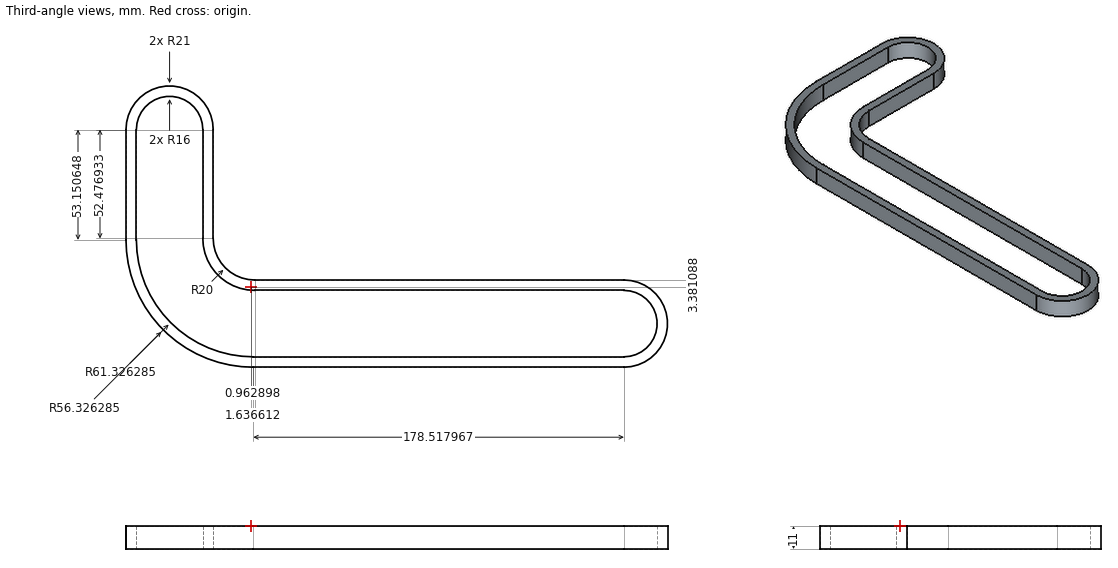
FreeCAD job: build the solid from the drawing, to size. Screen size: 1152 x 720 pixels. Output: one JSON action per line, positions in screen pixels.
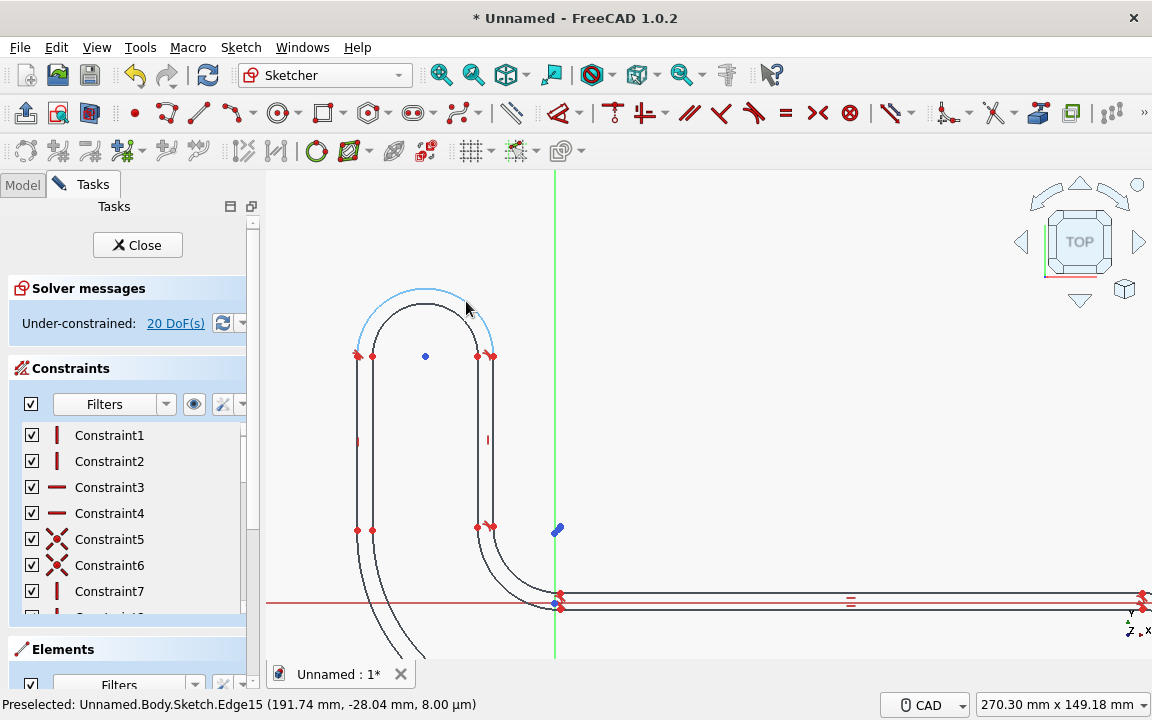
{"action": "left_click", "coordinate": [465, 302]}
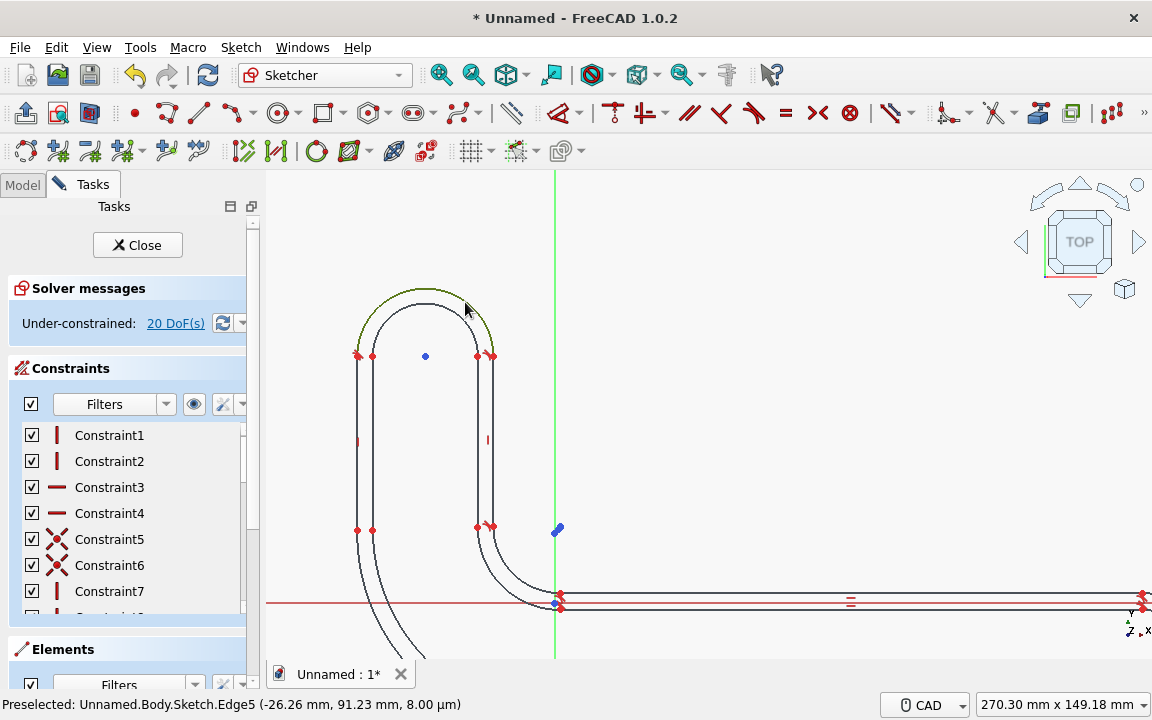
{"action": "left_click", "coordinate": [456, 314]}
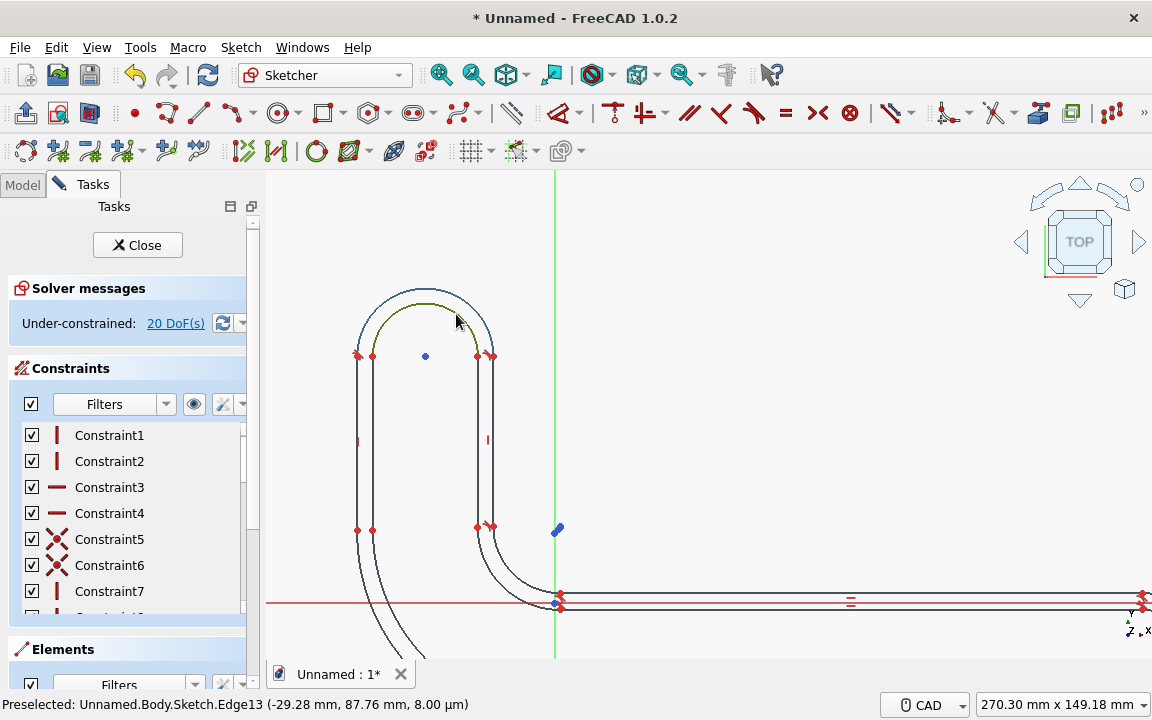
{"action": "left_click", "coordinate": [614, 114]}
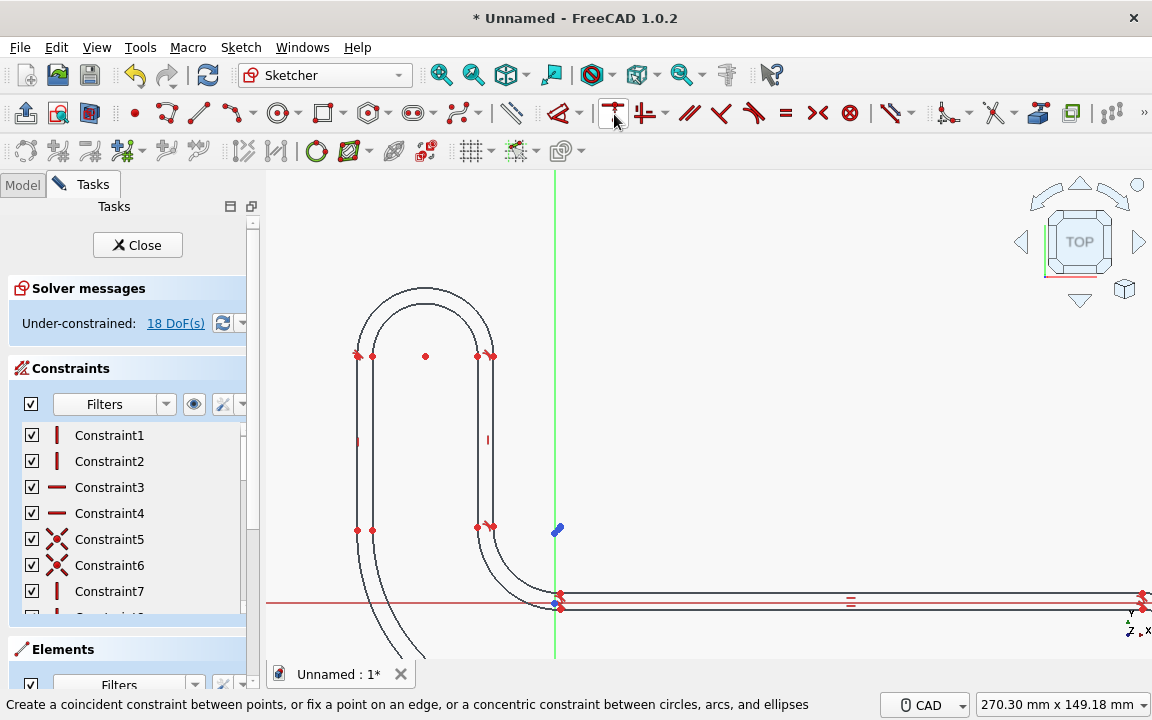
{"action": "left_click", "coordinate": [501, 557]}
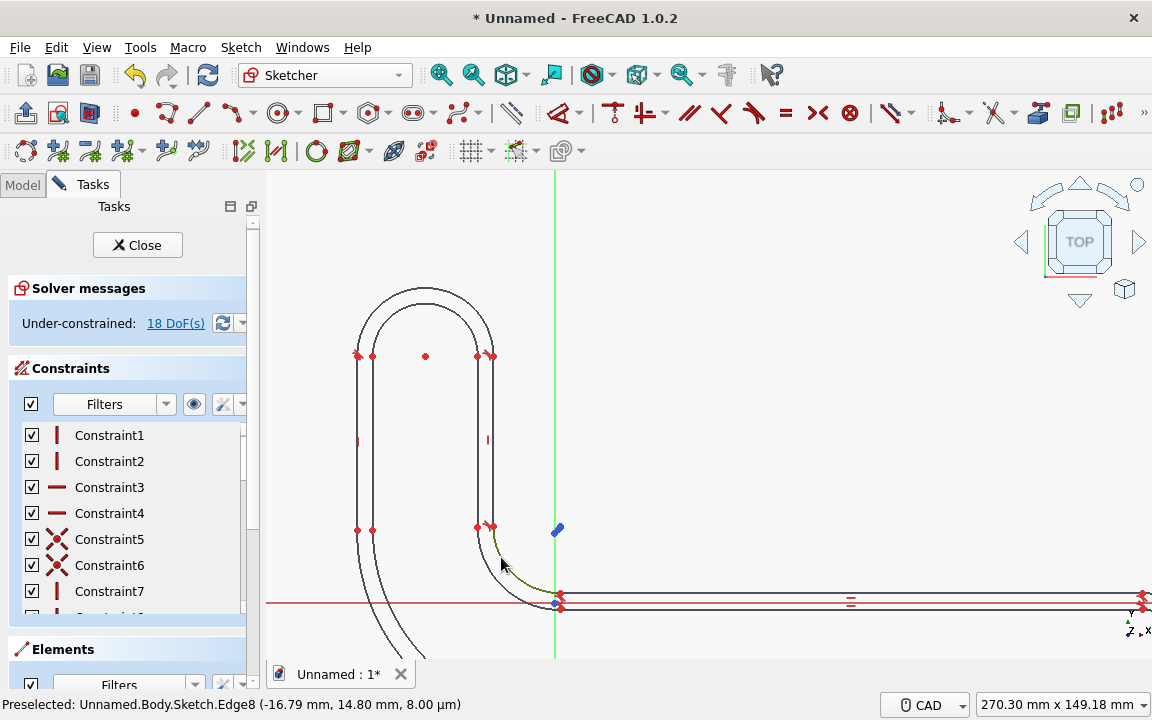
{"action": "left_click", "coordinate": [487, 565]}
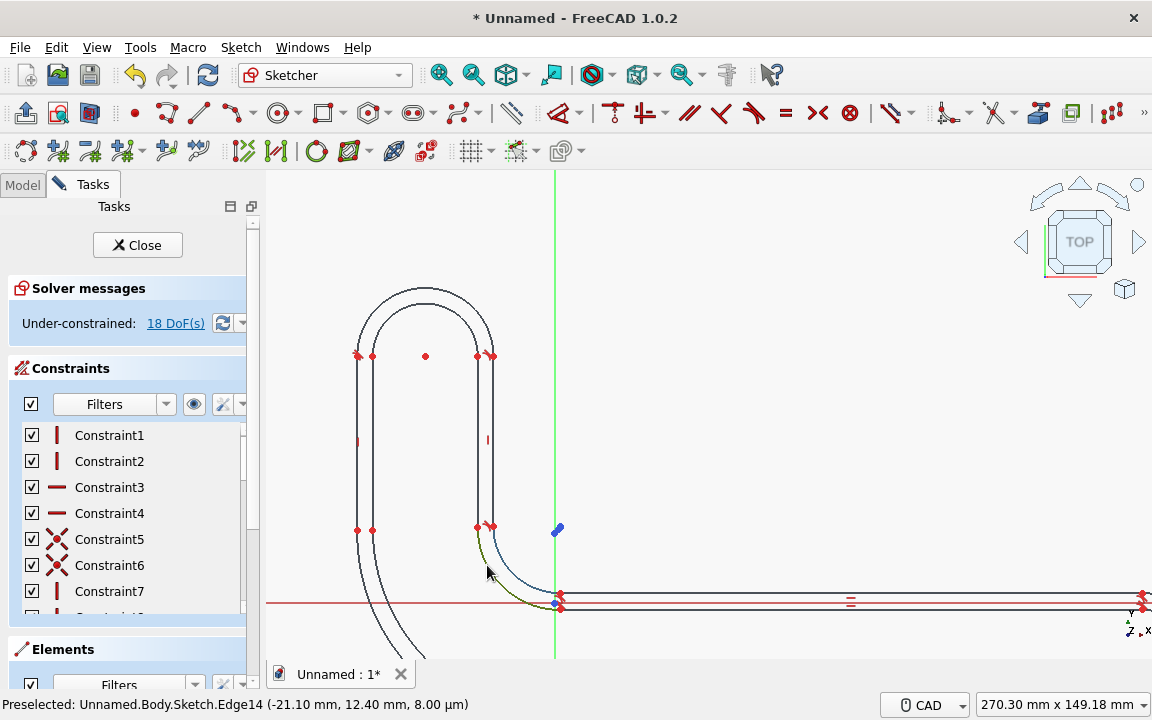
{"action": "left_click", "coordinate": [614, 114]}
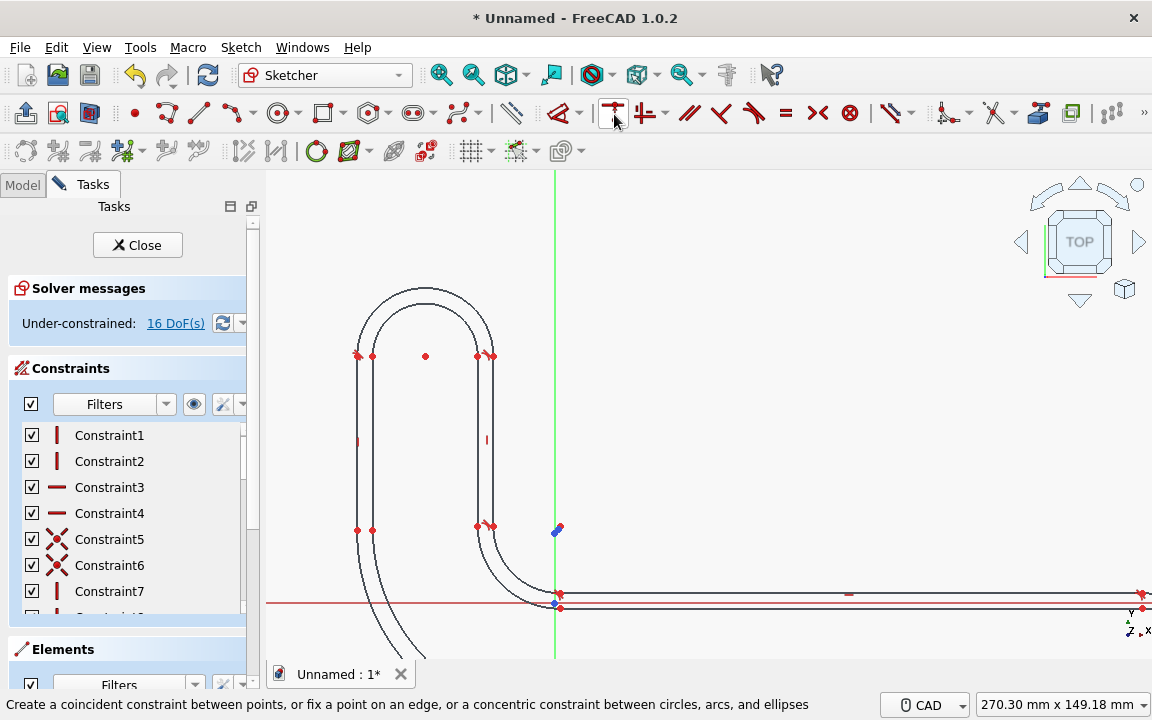
{"action": "scroll", "coordinate": [465, 301], "scroll_direction": "down", "scroll_amount": 3}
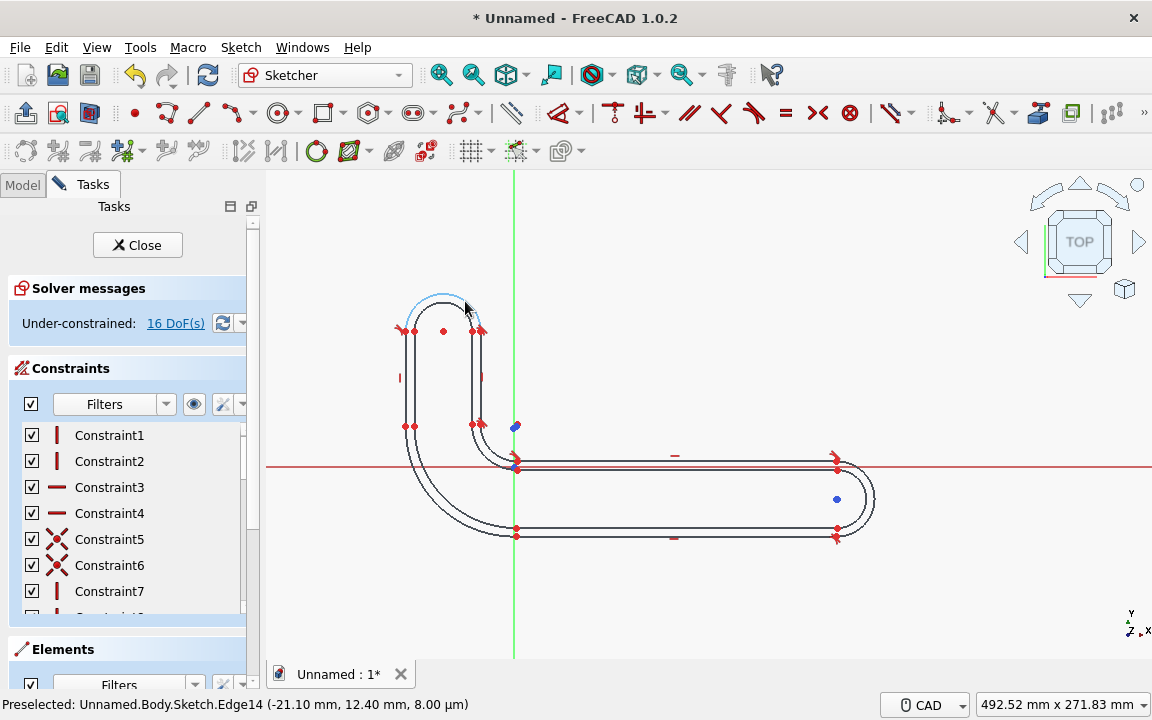
{"action": "scroll", "coordinate": [867, 521], "scroll_direction": "up", "scroll_amount": 3}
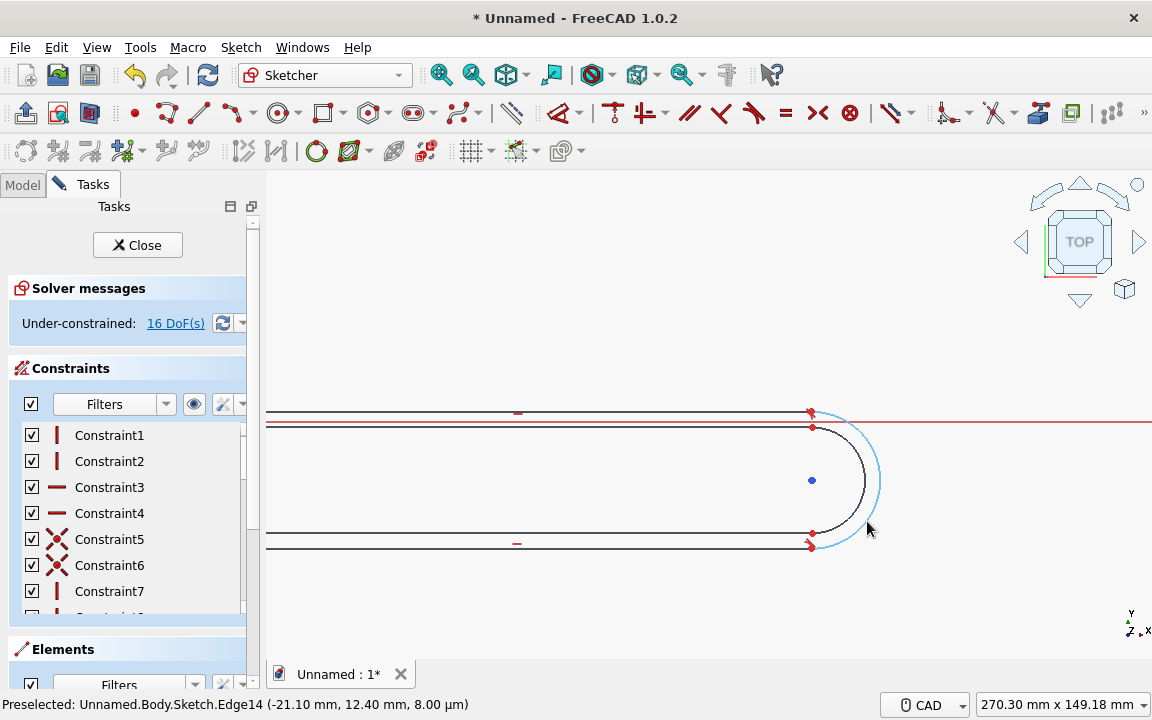
{"action": "left_click", "coordinate": [867, 521]}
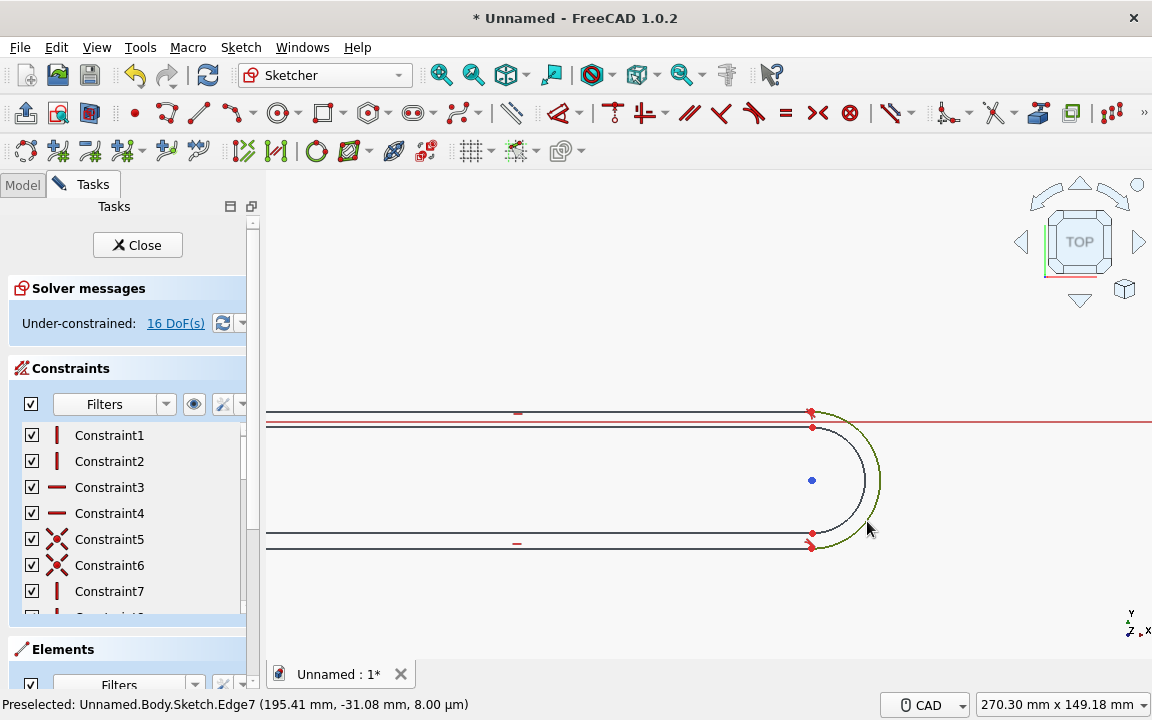
{"action": "left_click", "coordinate": [855, 511]}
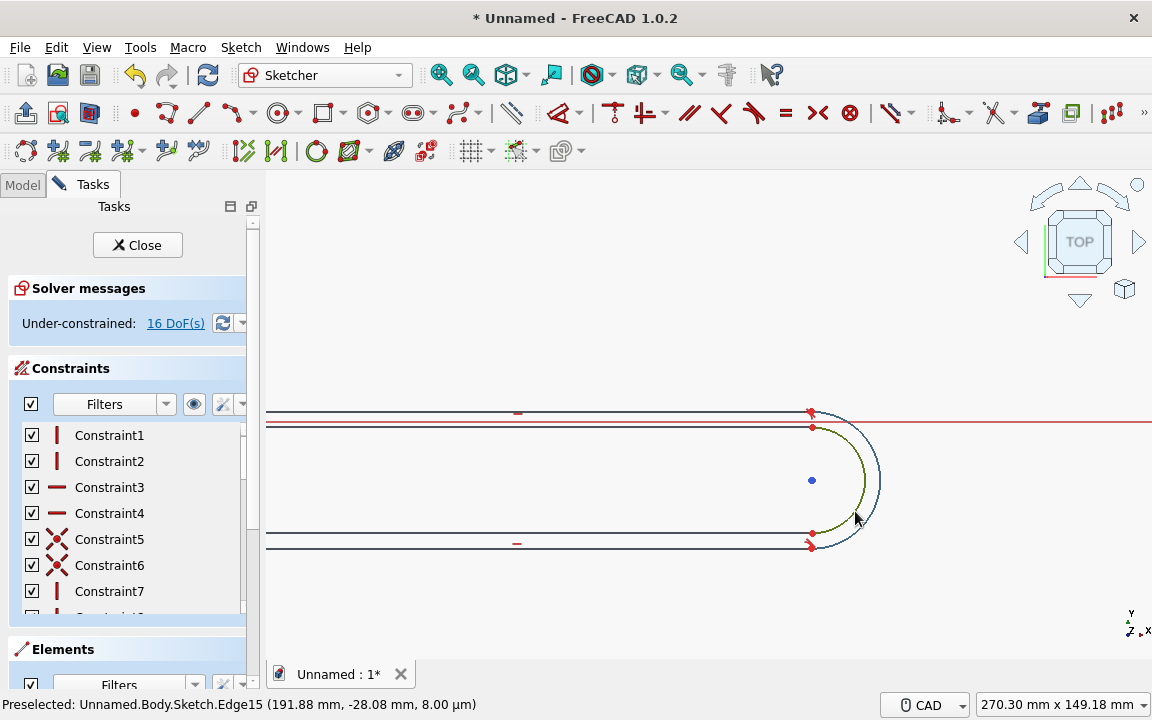
{"action": "left_click", "coordinate": [614, 114]}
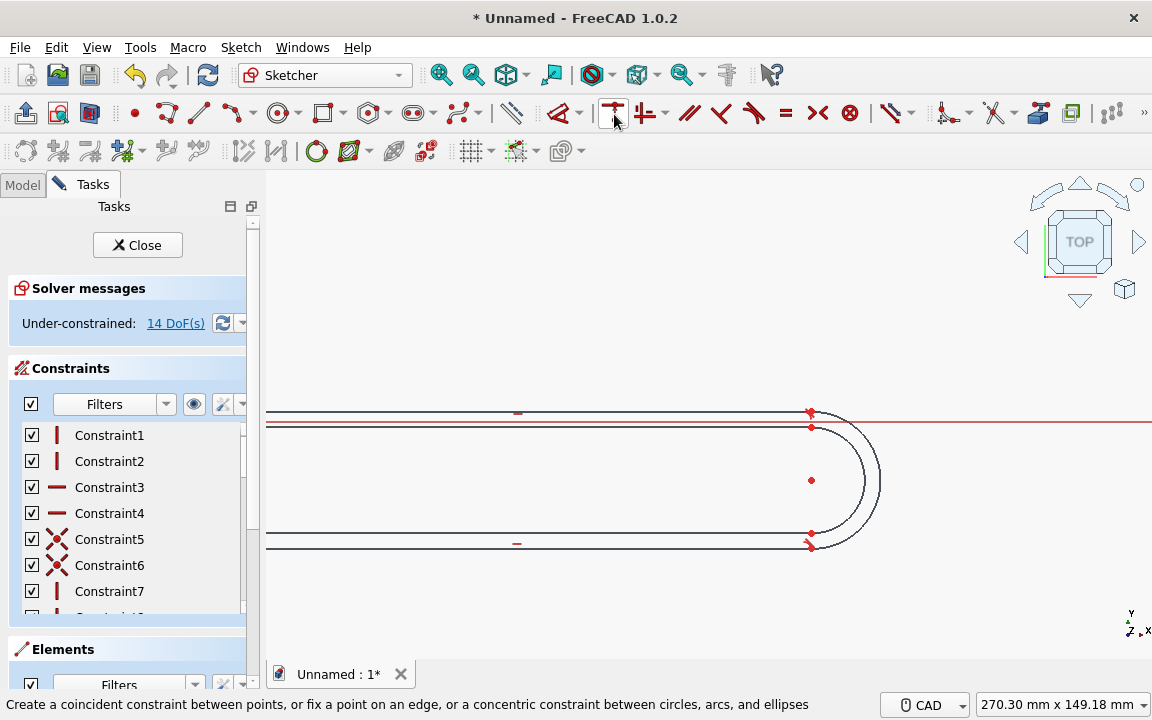
{"action": "scroll", "coordinate": [868, 521], "scroll_direction": "down", "scroll_amount": 3}